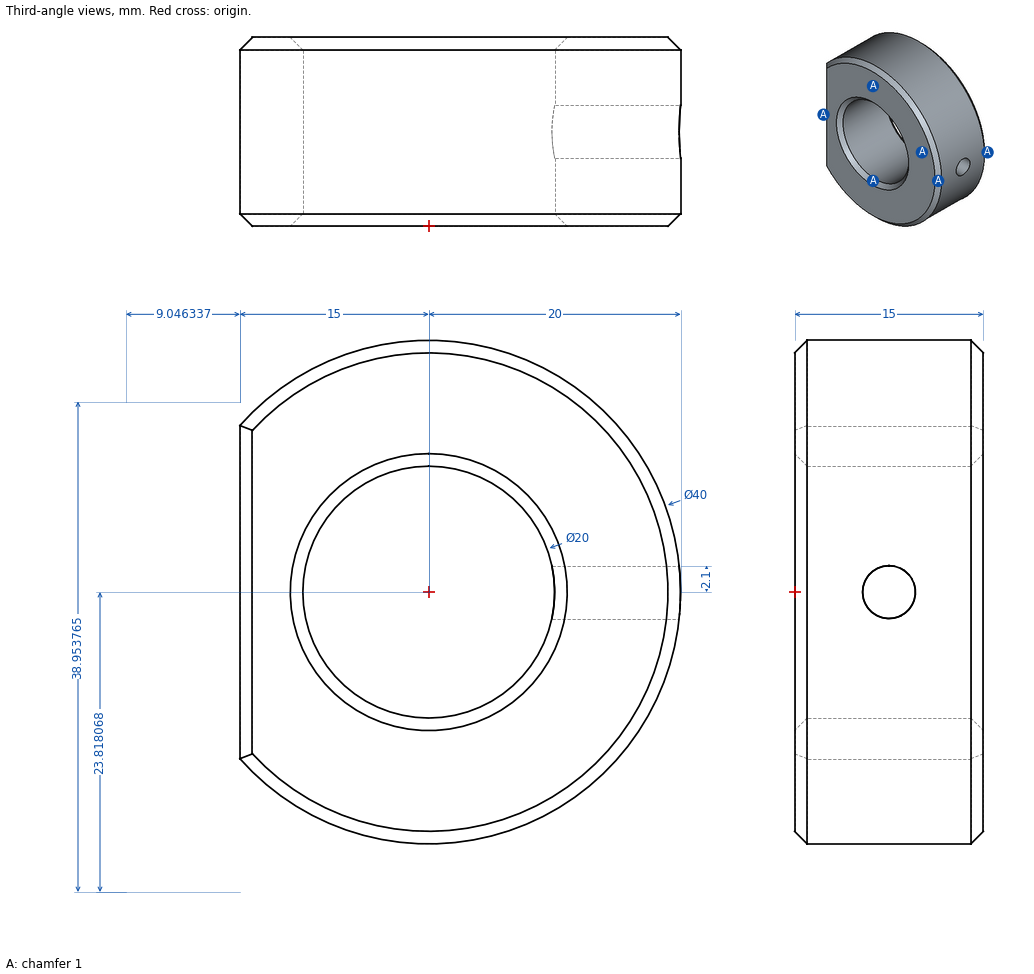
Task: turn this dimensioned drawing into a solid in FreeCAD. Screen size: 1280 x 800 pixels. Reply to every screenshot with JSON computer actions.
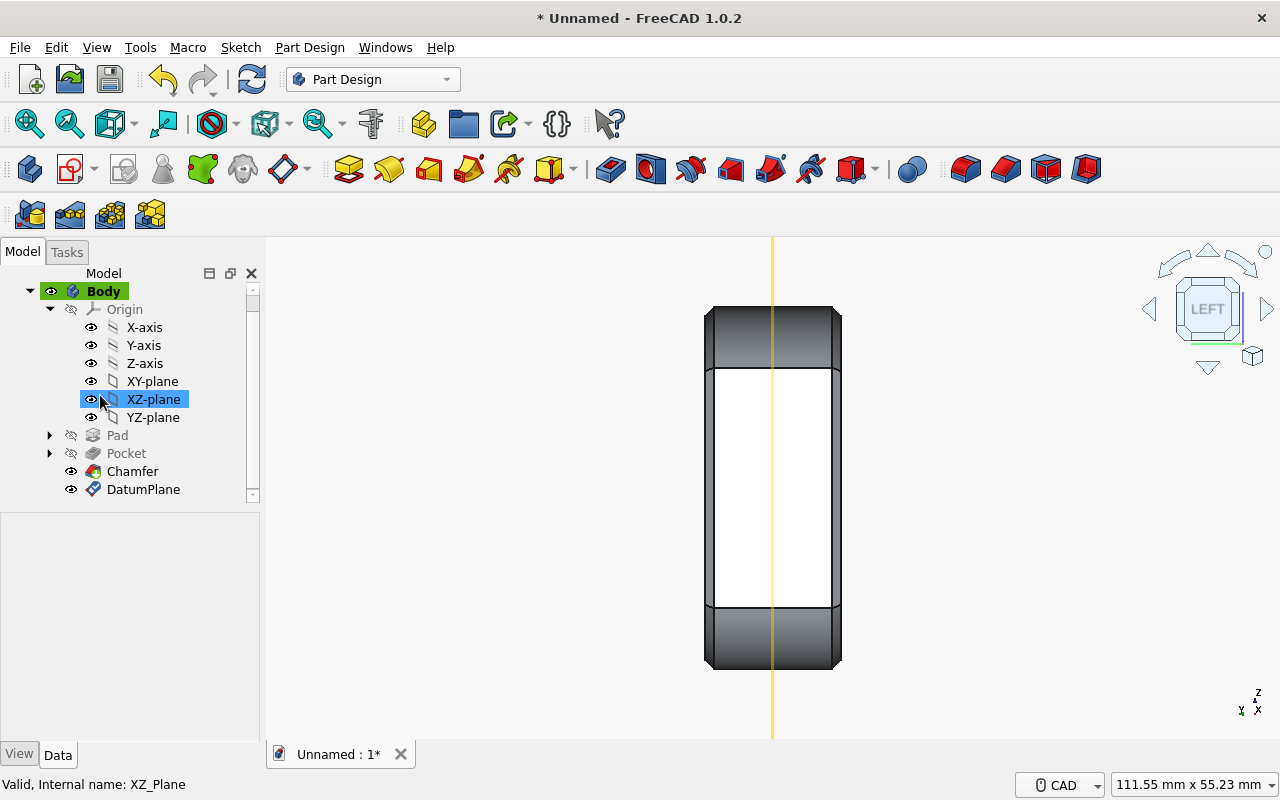
{"action": "left_click", "coordinate": [116, 489]}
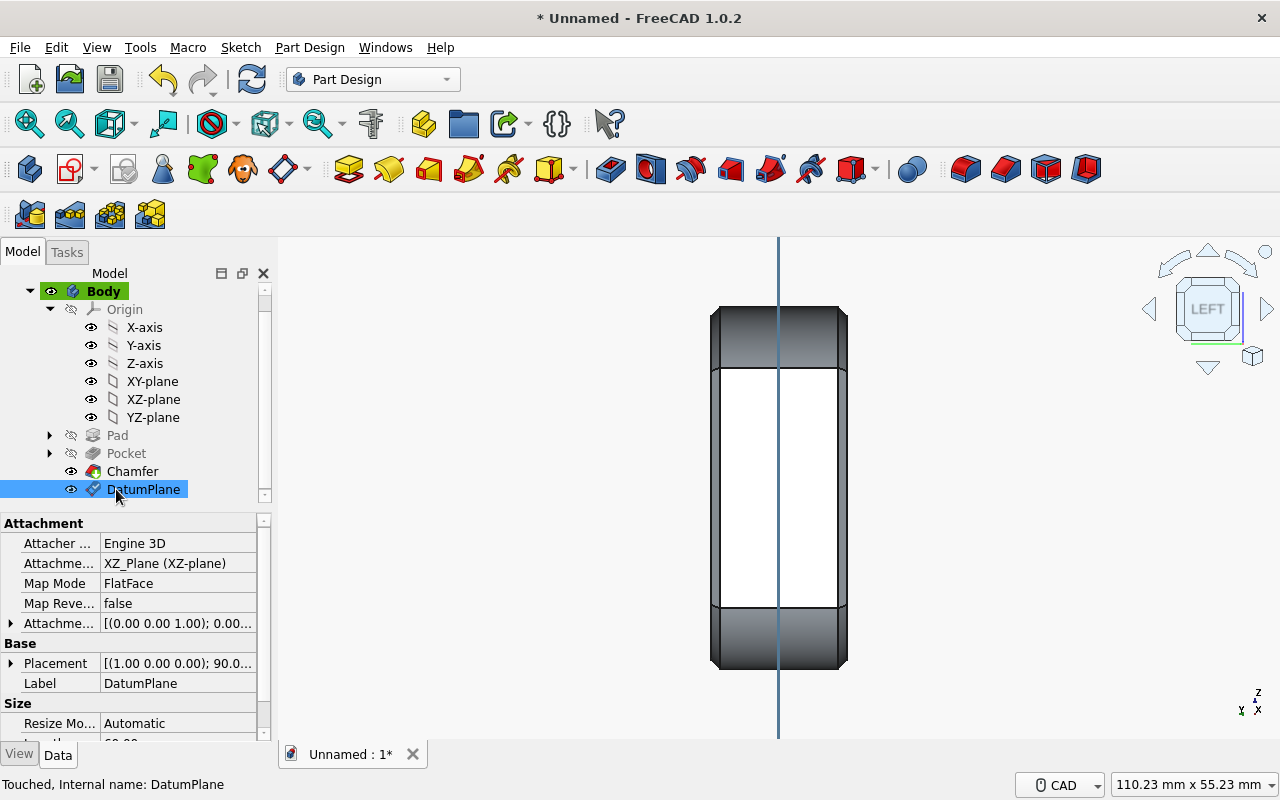
{"action": "left_click", "coordinate": [70, 170]}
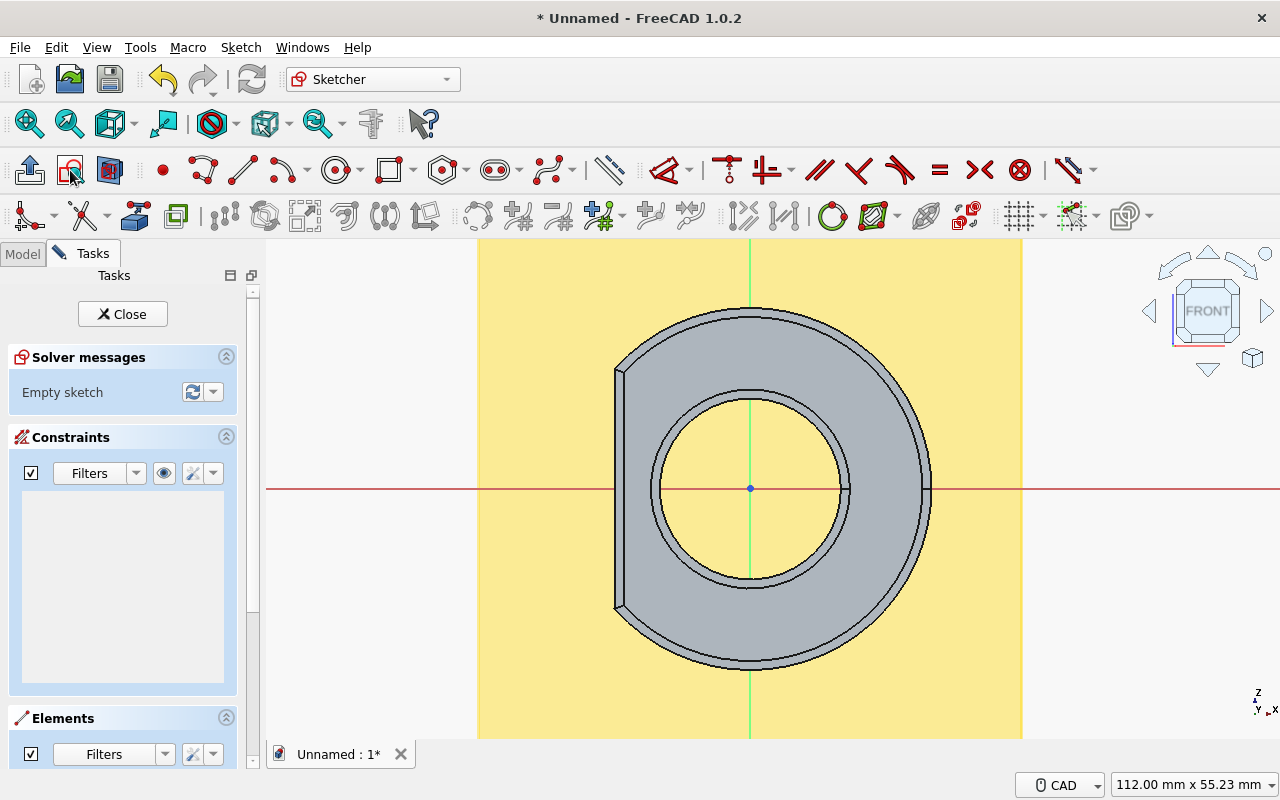
{"action": "left_click", "coordinate": [110, 170]}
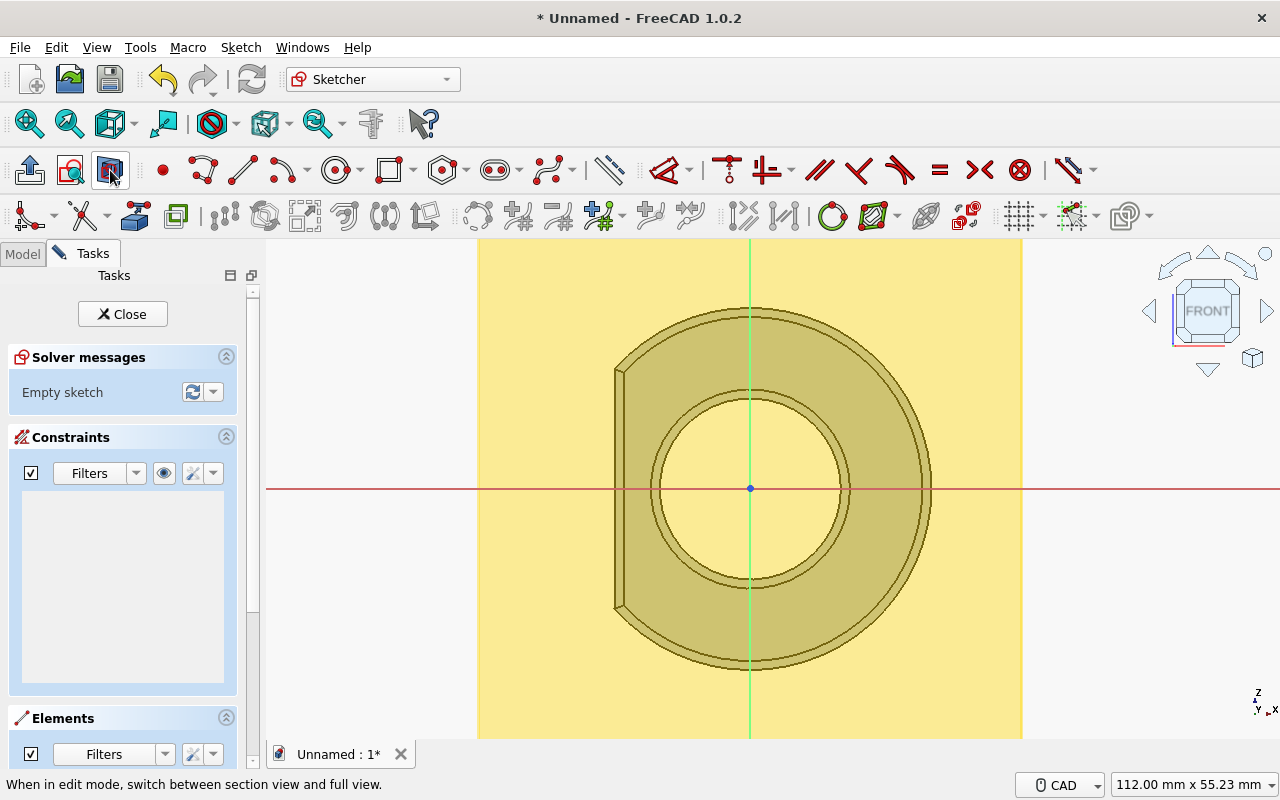
{"action": "scroll", "coordinate": [900, 475], "scroll_direction": "up", "scroll_amount": 6}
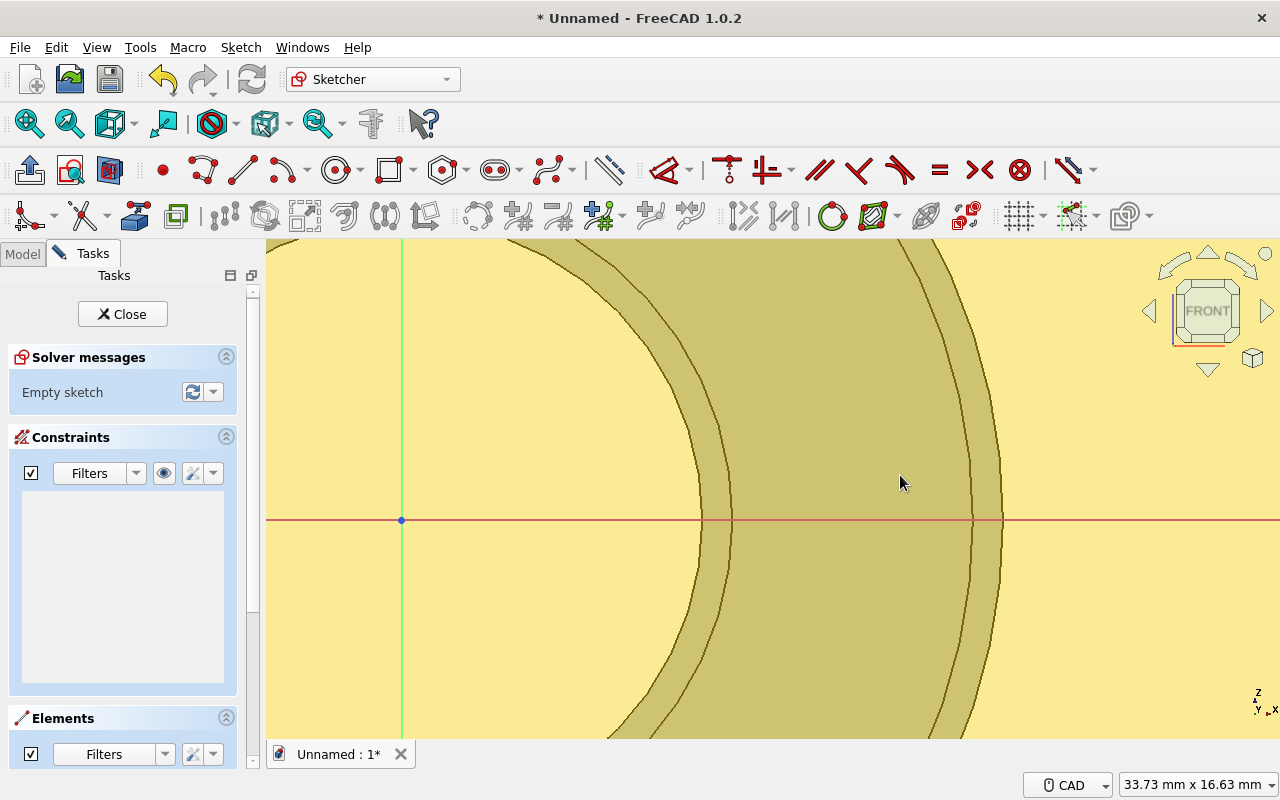
{"action": "left_click", "coordinate": [390, 170]}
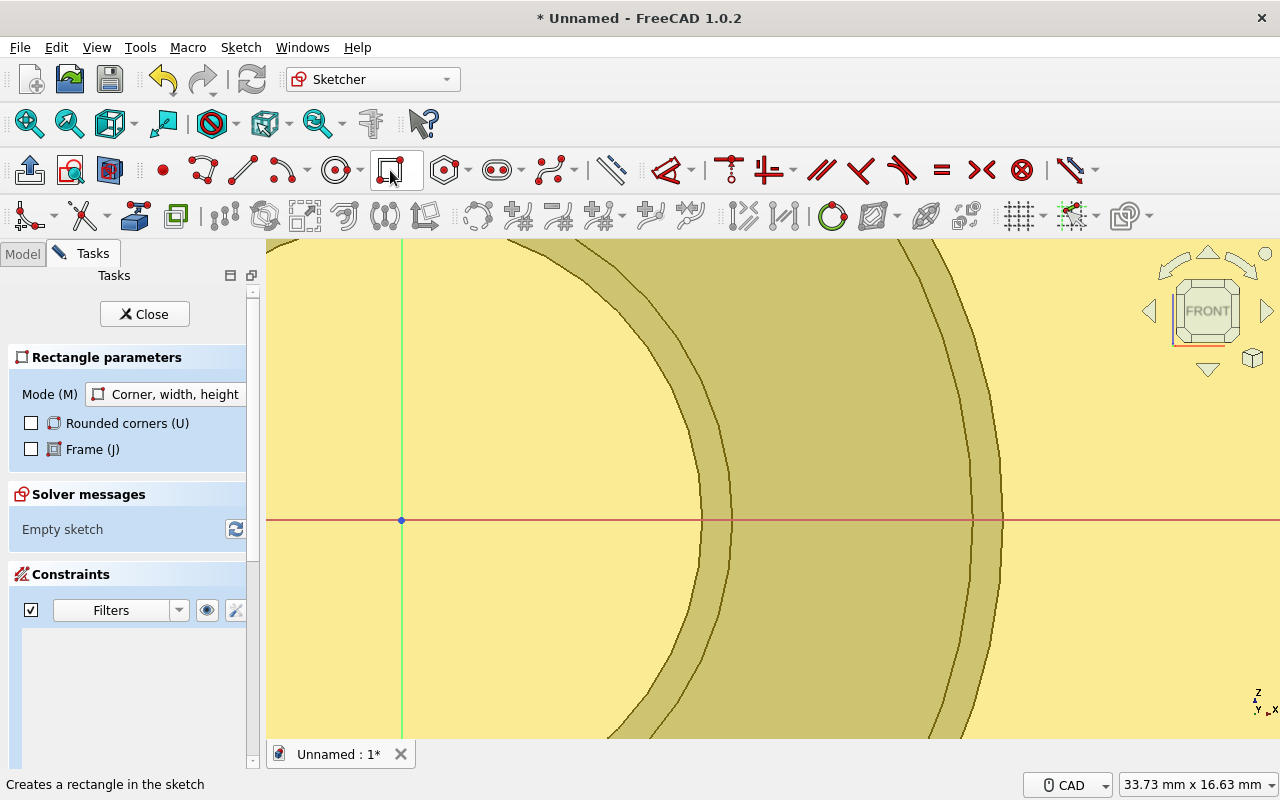
{"action": "left_click", "coordinate": [402, 520]}
{"action": "mouse_move", "coordinate": [1003, 457]}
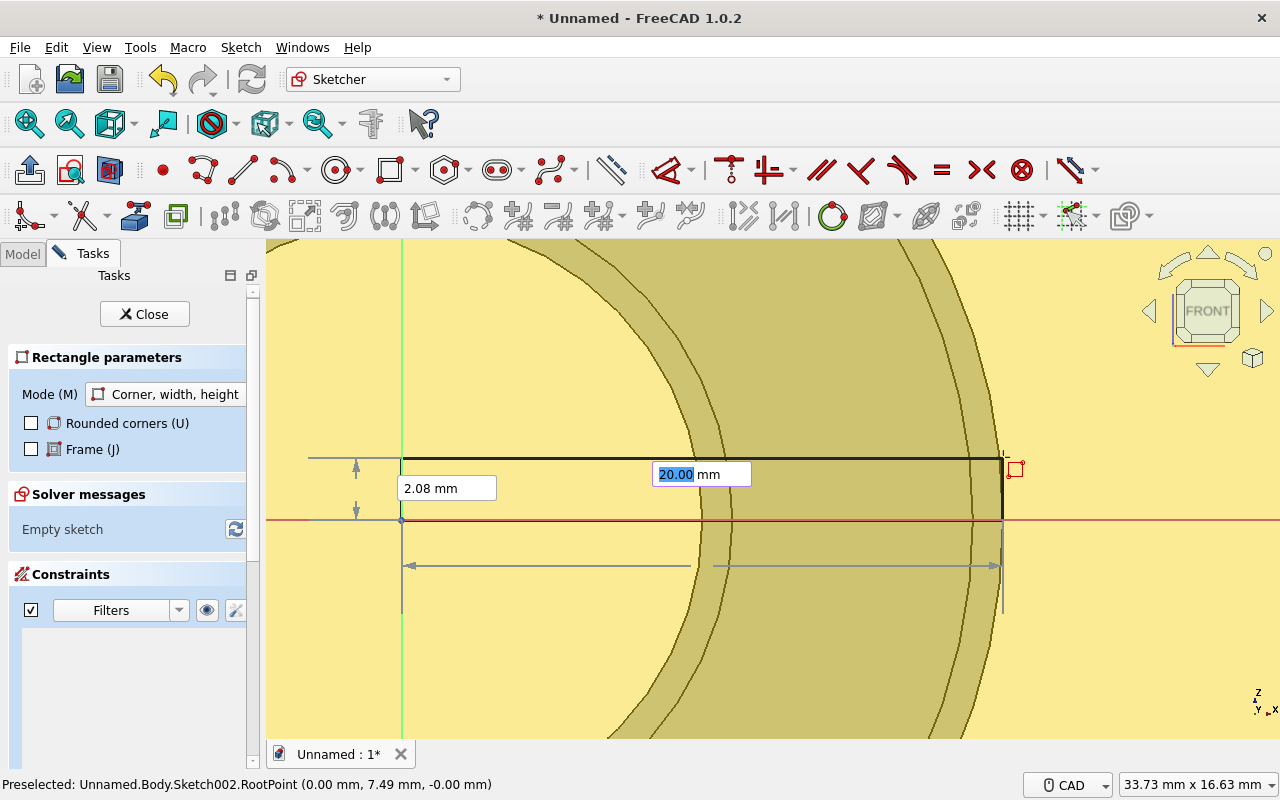
{"action": "type", "text": "20"}
{"action": "key", "text": "Tab"}
{"action": "type", "text": "2.1"}
{"action": "key", "text": "Return"}
{"action": "key", "text": "Escape"}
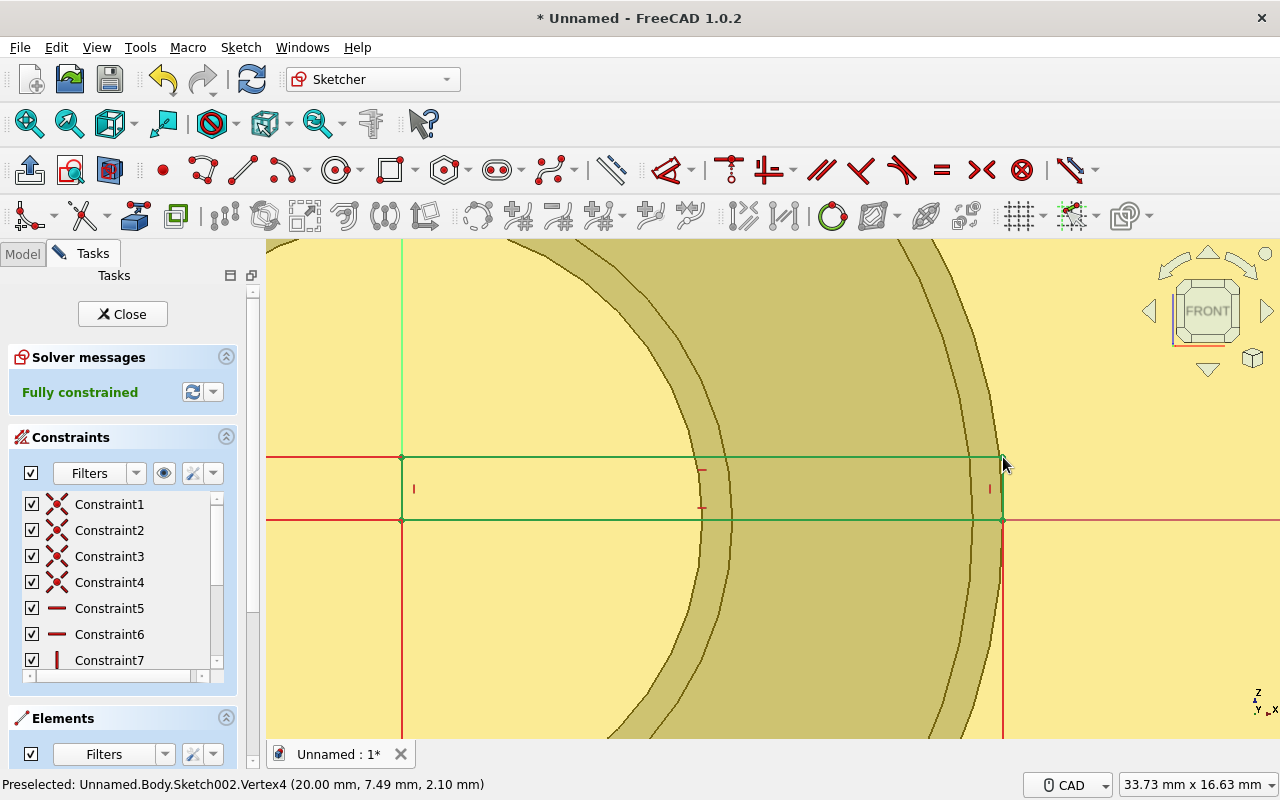
{"action": "left_click", "coordinate": [123, 314]}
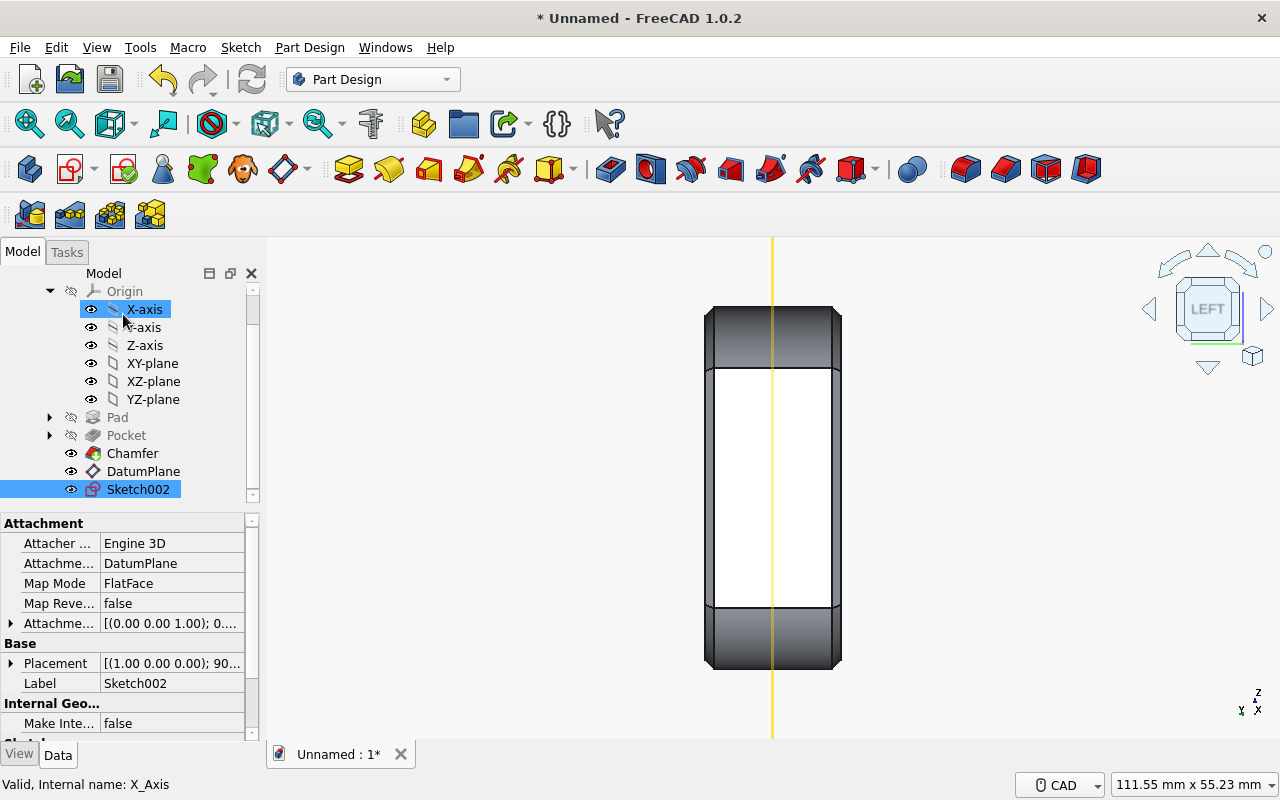
{"action": "left_click", "coordinate": [692, 170]}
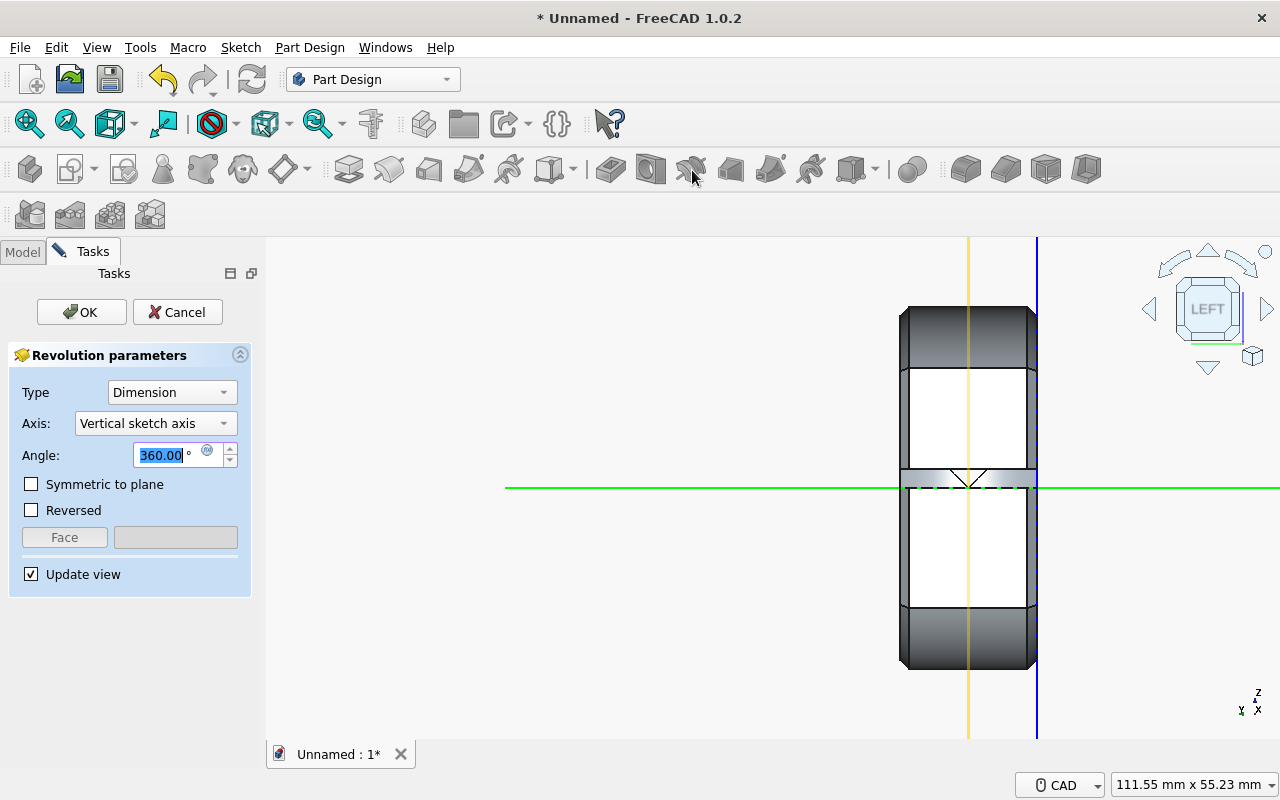
{"action": "left_click", "coordinate": [156, 424]}